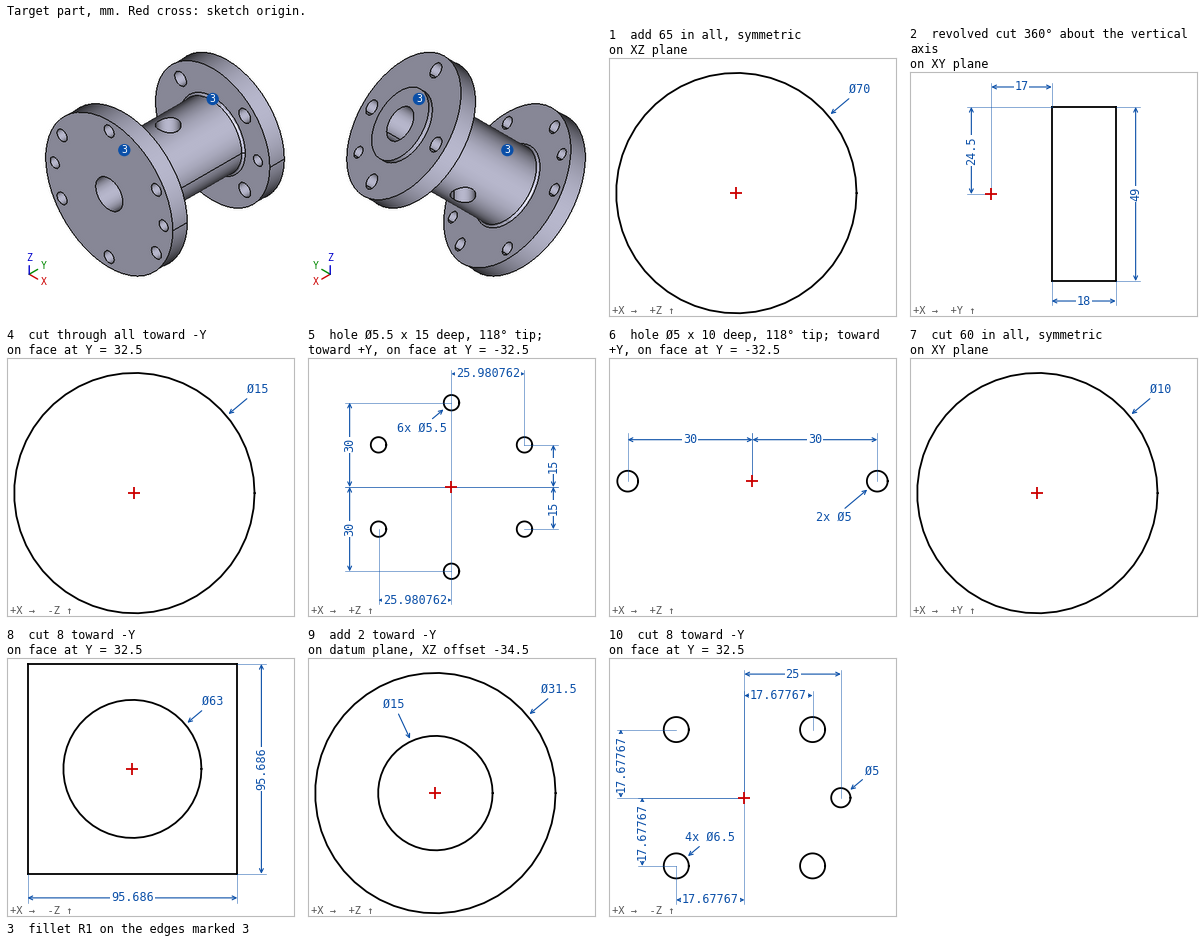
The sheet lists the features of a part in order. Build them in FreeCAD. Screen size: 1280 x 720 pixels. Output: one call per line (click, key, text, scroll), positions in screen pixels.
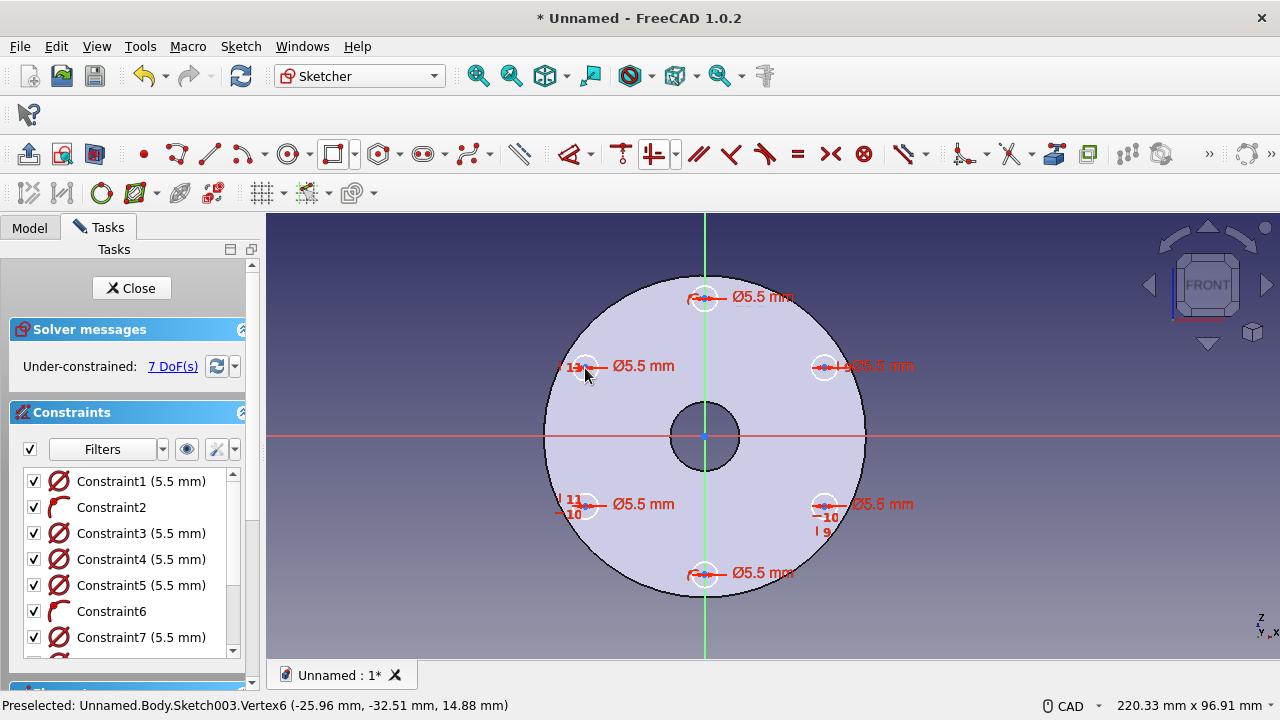
click(825, 368)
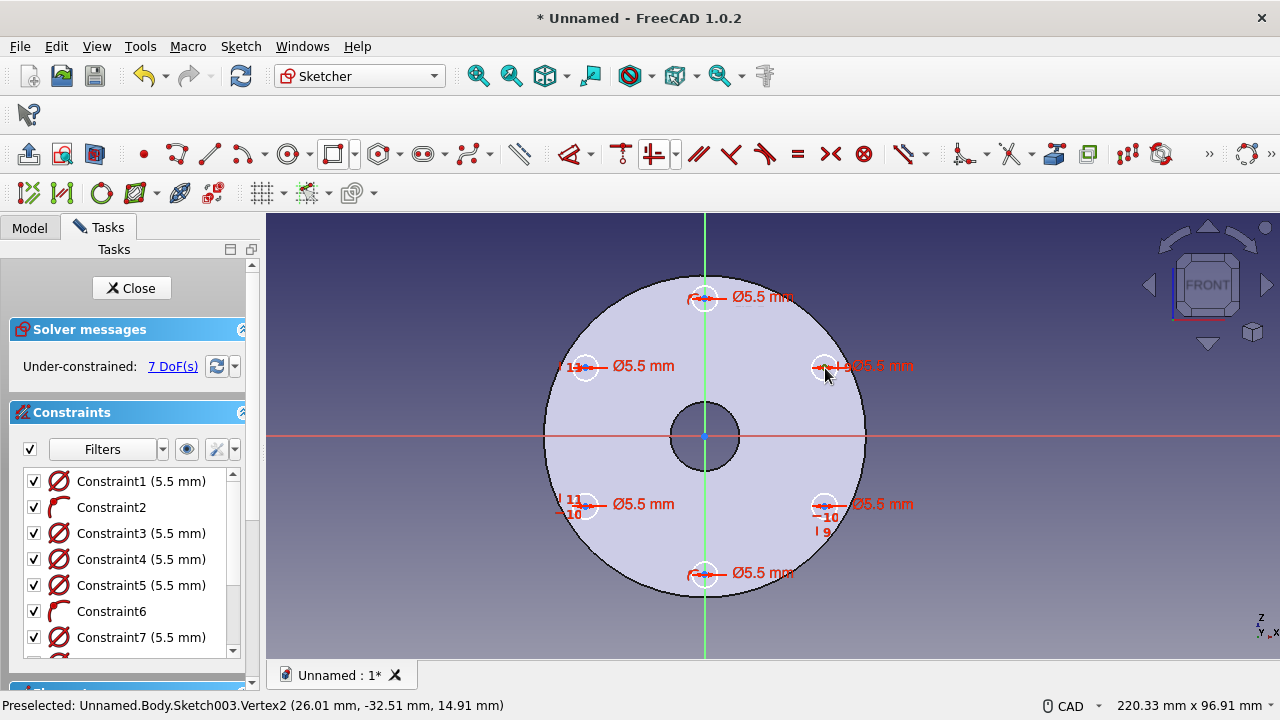
click(585, 368)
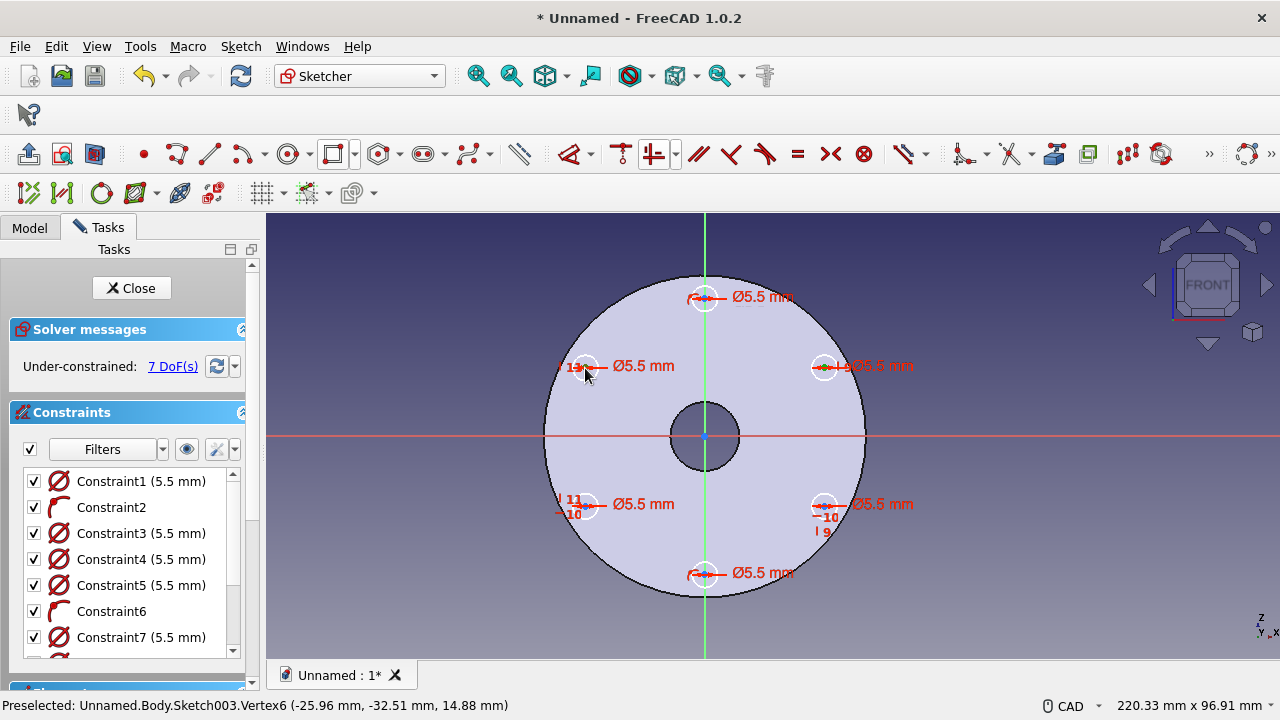
click(676, 154)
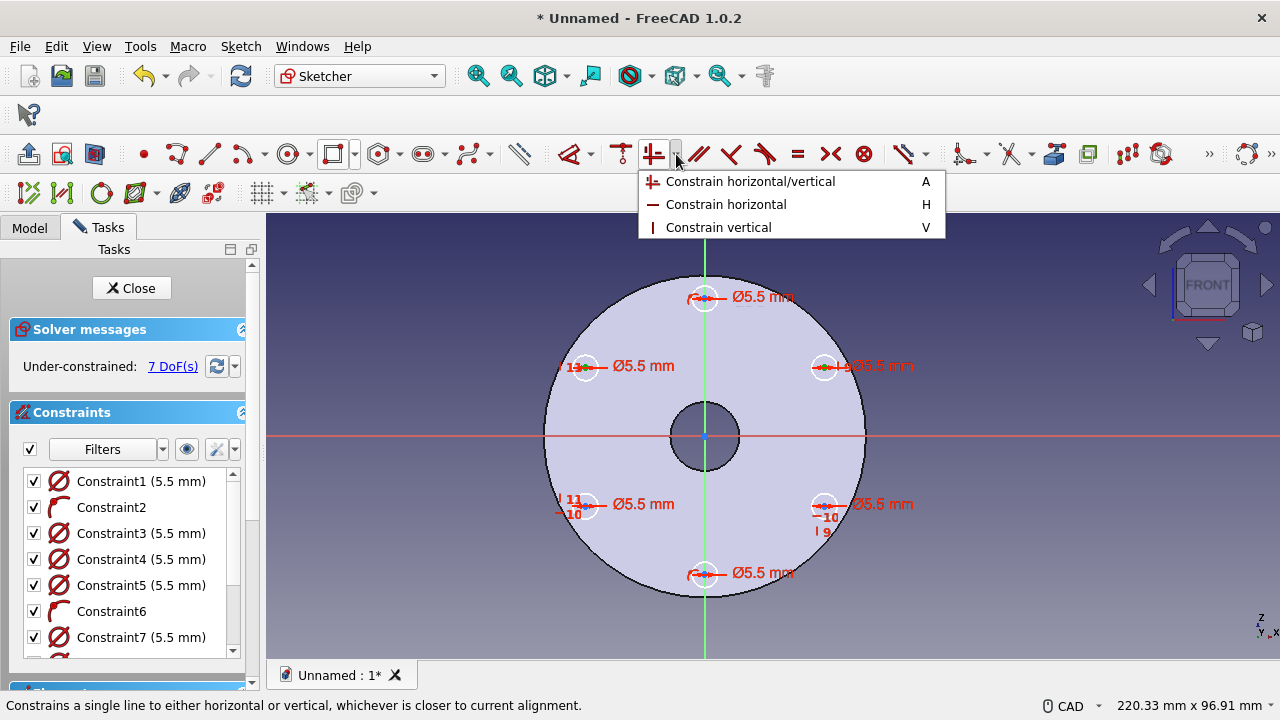
click(792, 204)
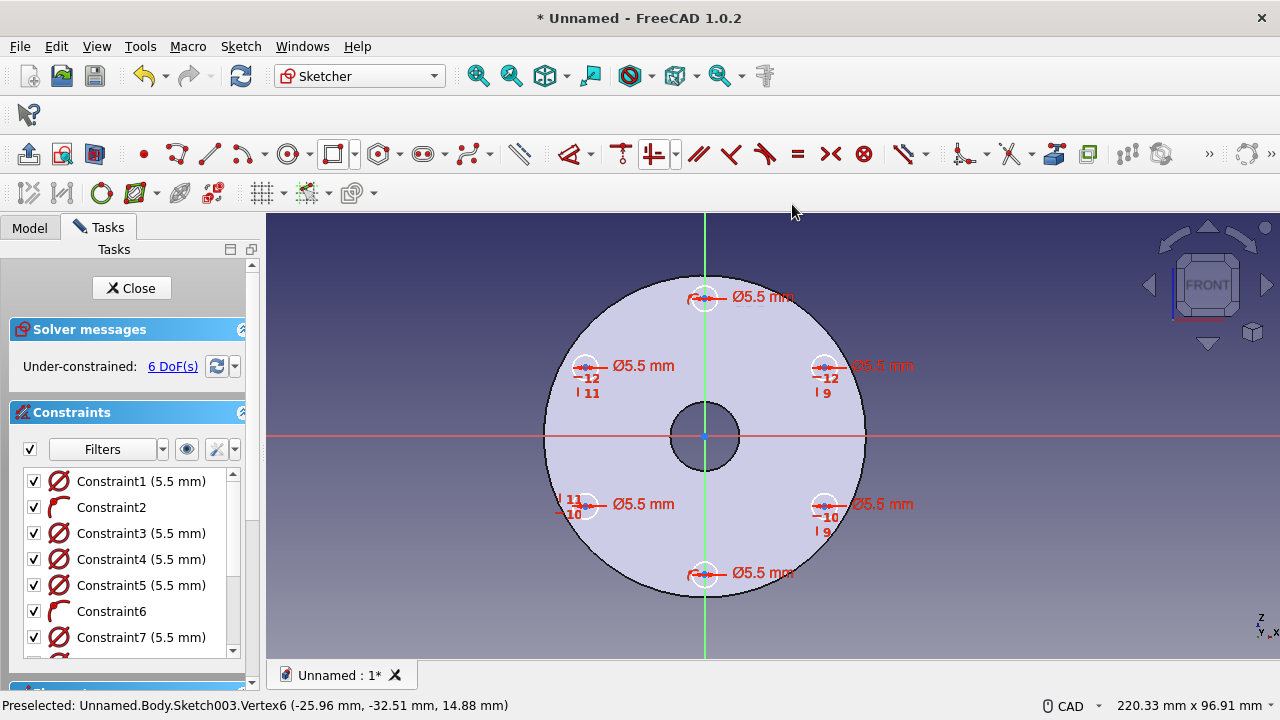
click(568, 154)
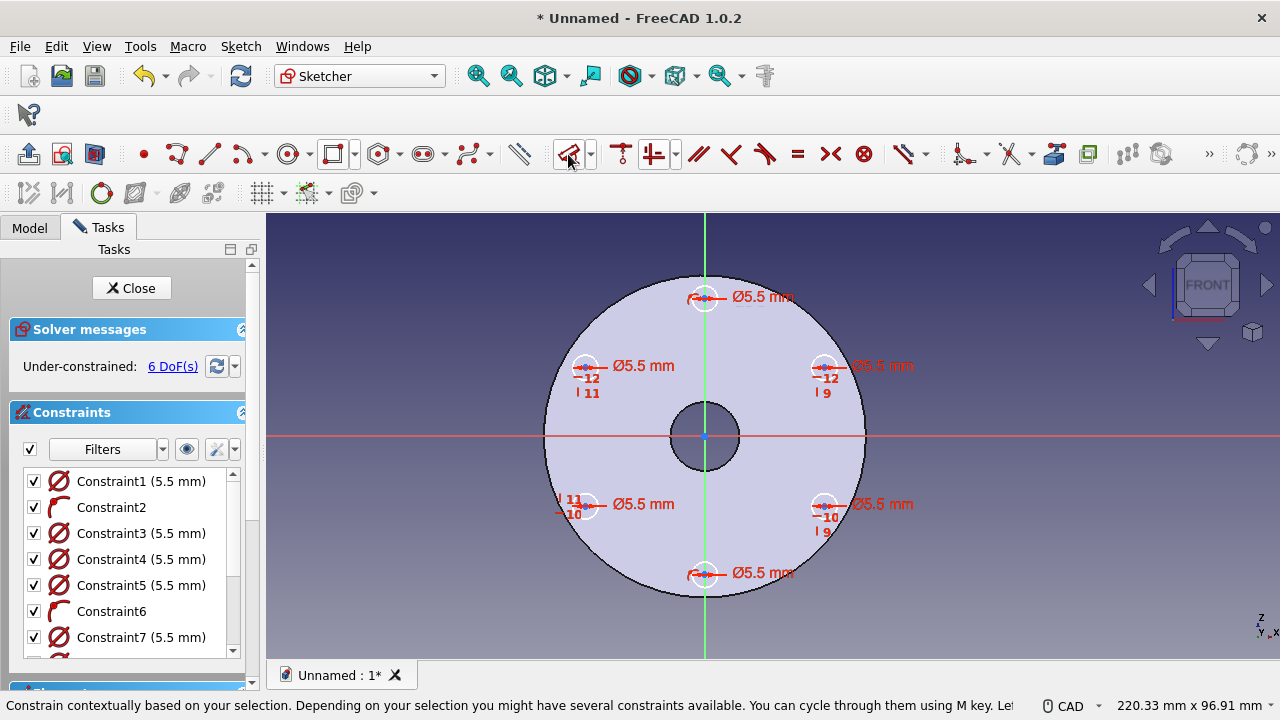
click(705, 299)
click(739, 368)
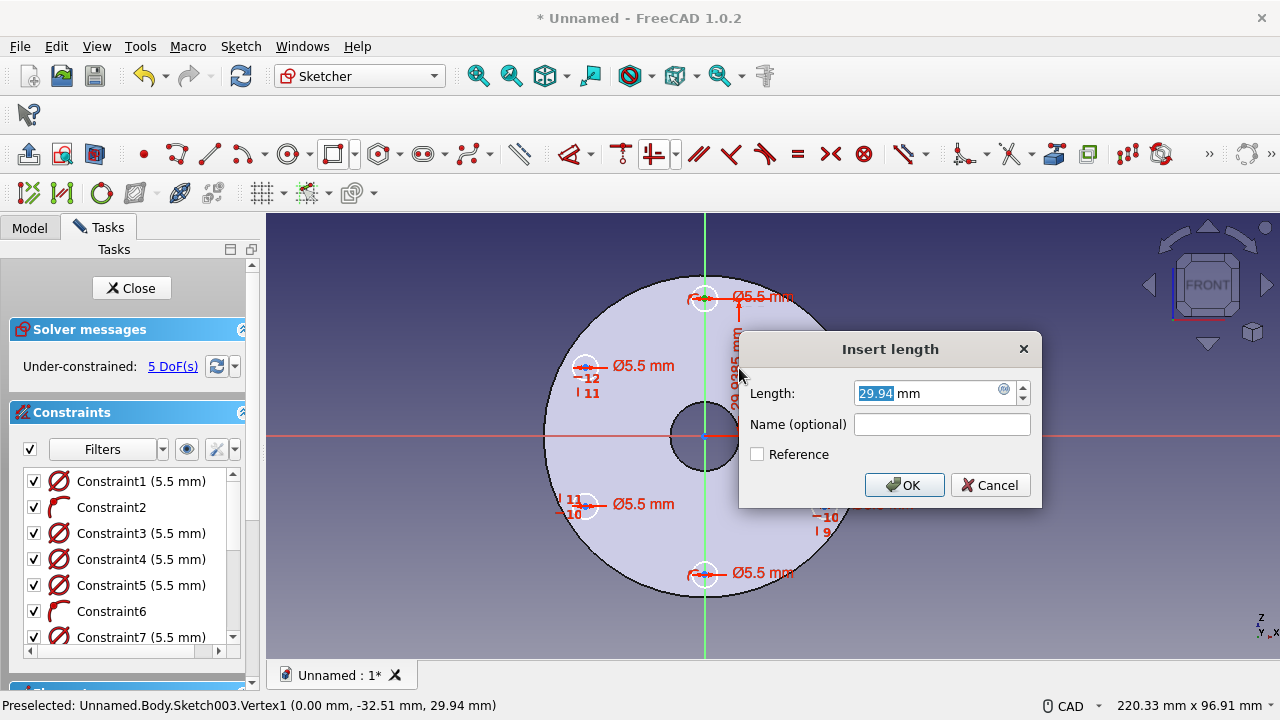
text(30)
key(Return)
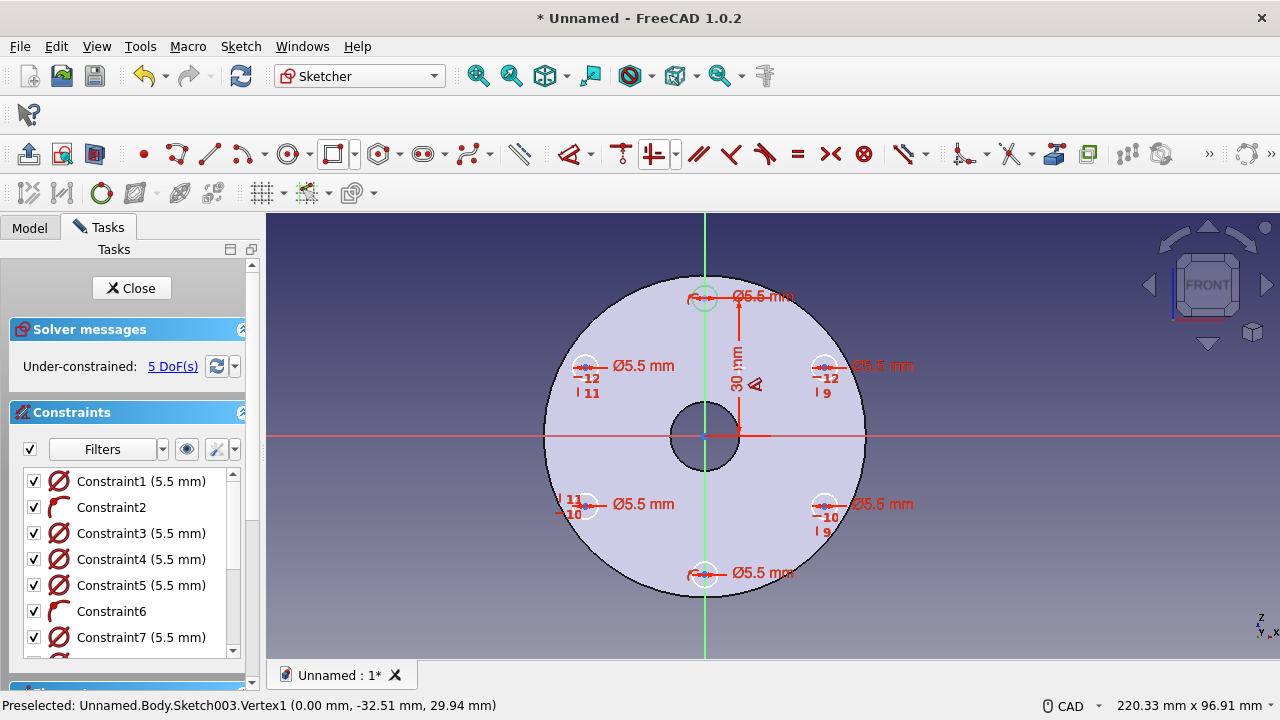
click(825, 368)
click(859, 402)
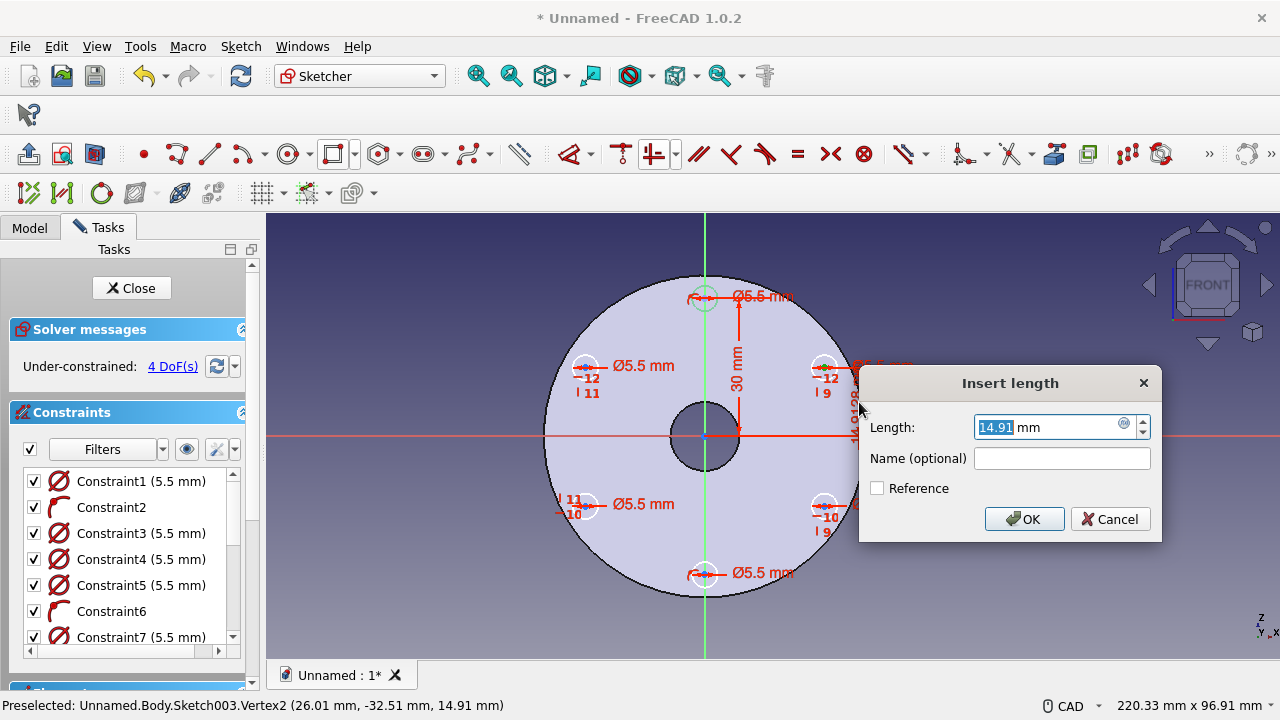
text(15)
key(Return)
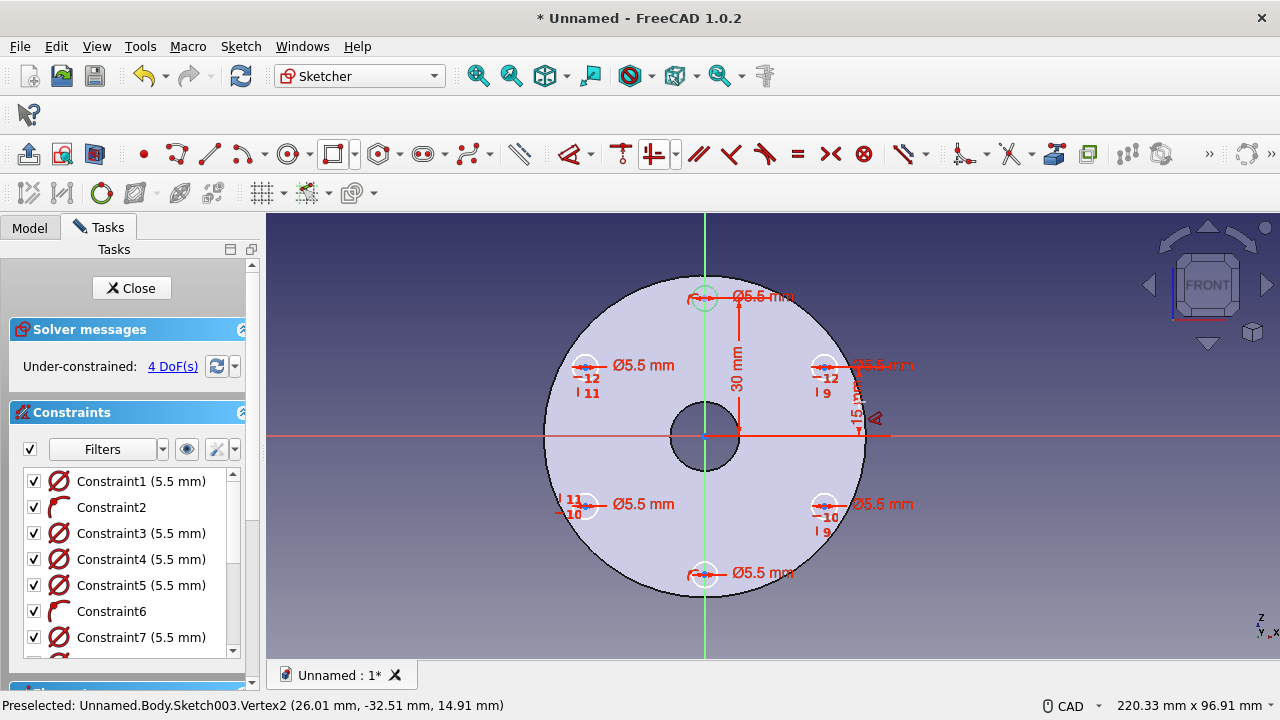
click(825, 506)
click(859, 471)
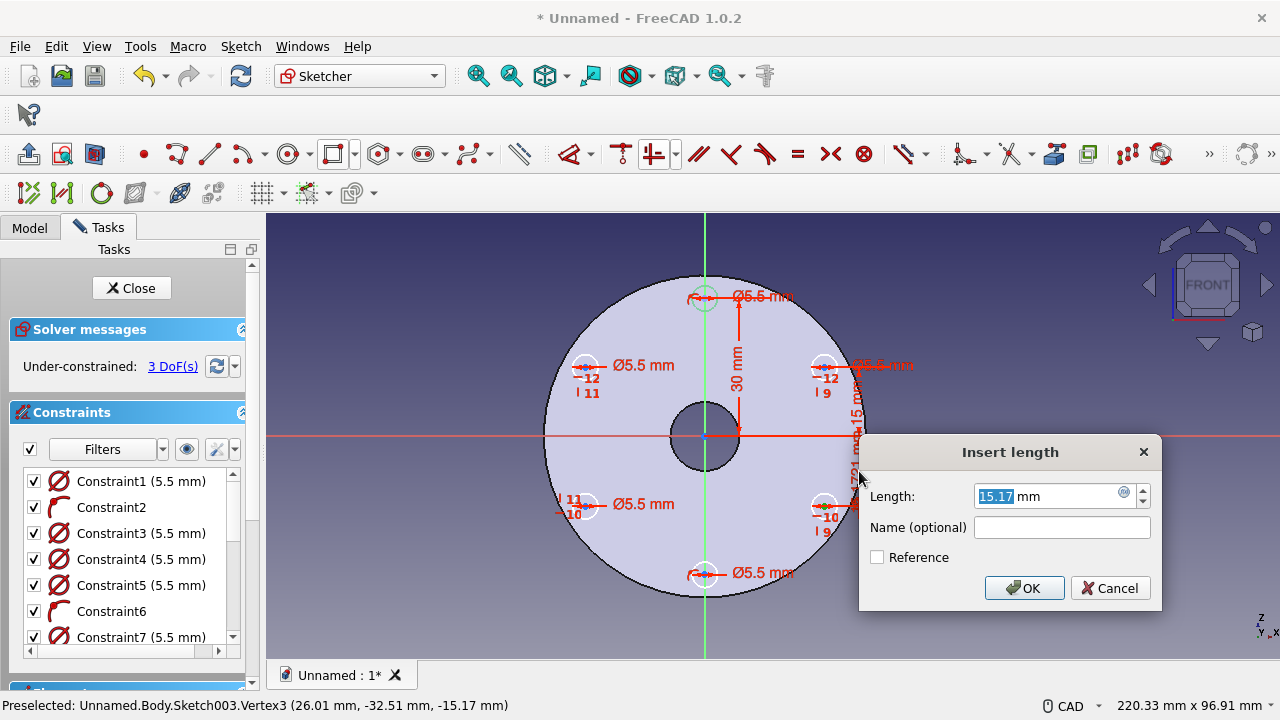
text(15)
key(Return)